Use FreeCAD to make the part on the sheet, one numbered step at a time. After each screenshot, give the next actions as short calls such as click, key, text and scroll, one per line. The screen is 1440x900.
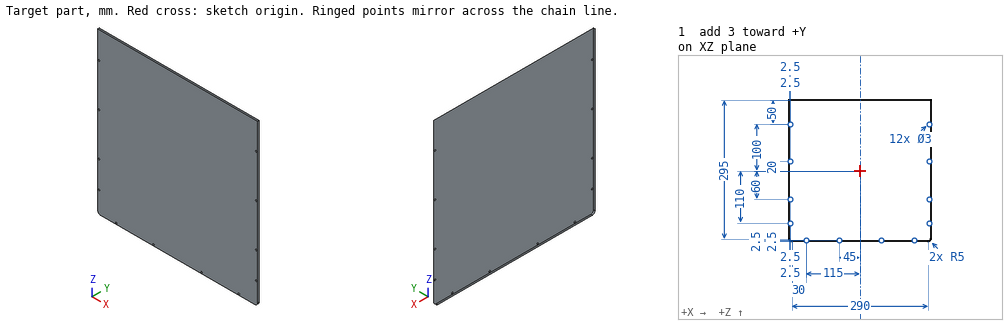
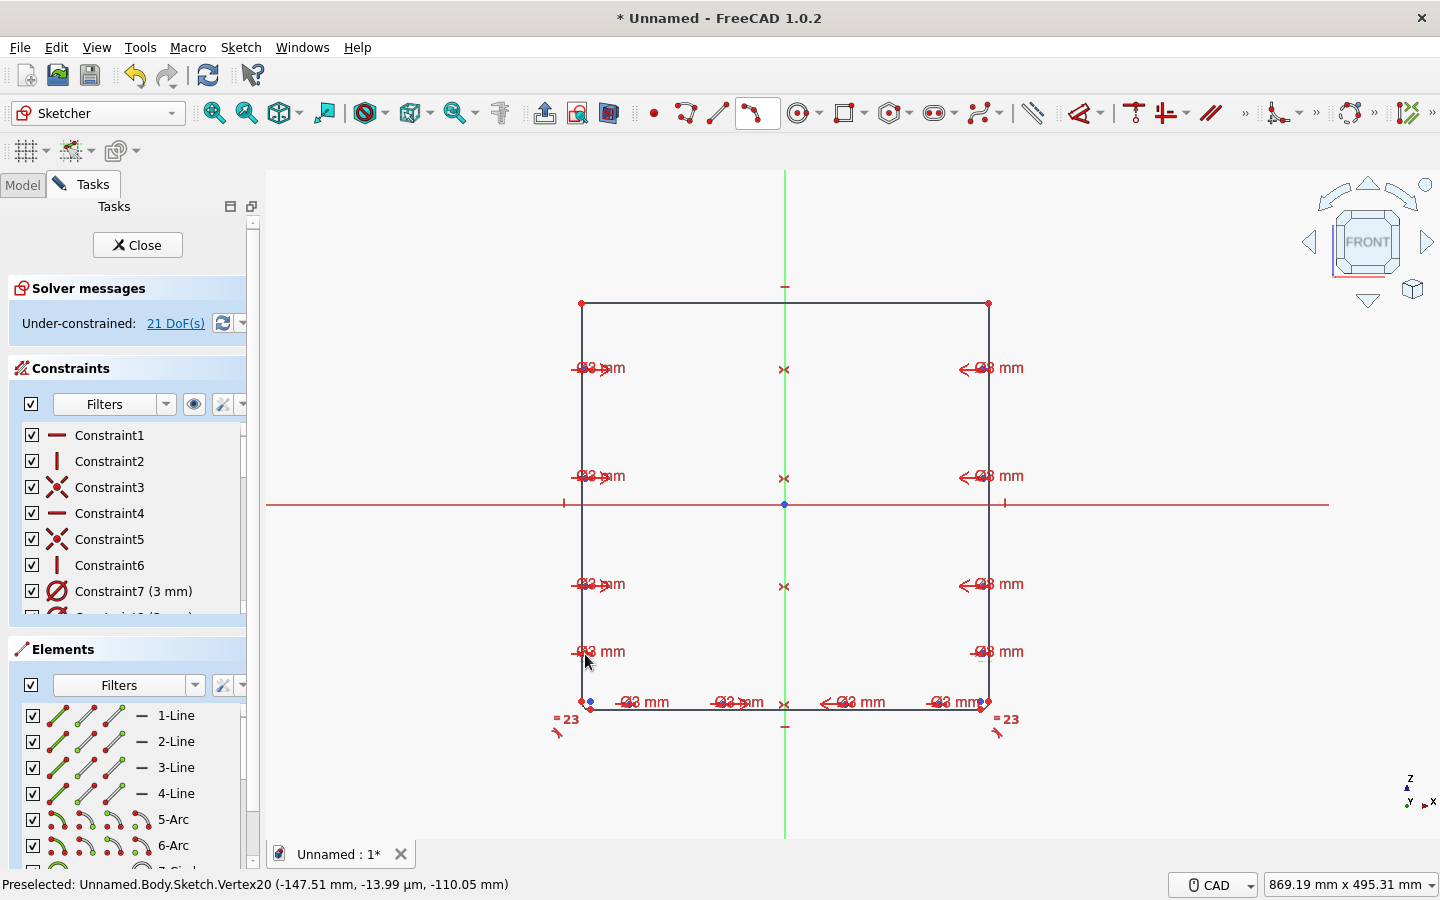
click(984, 654)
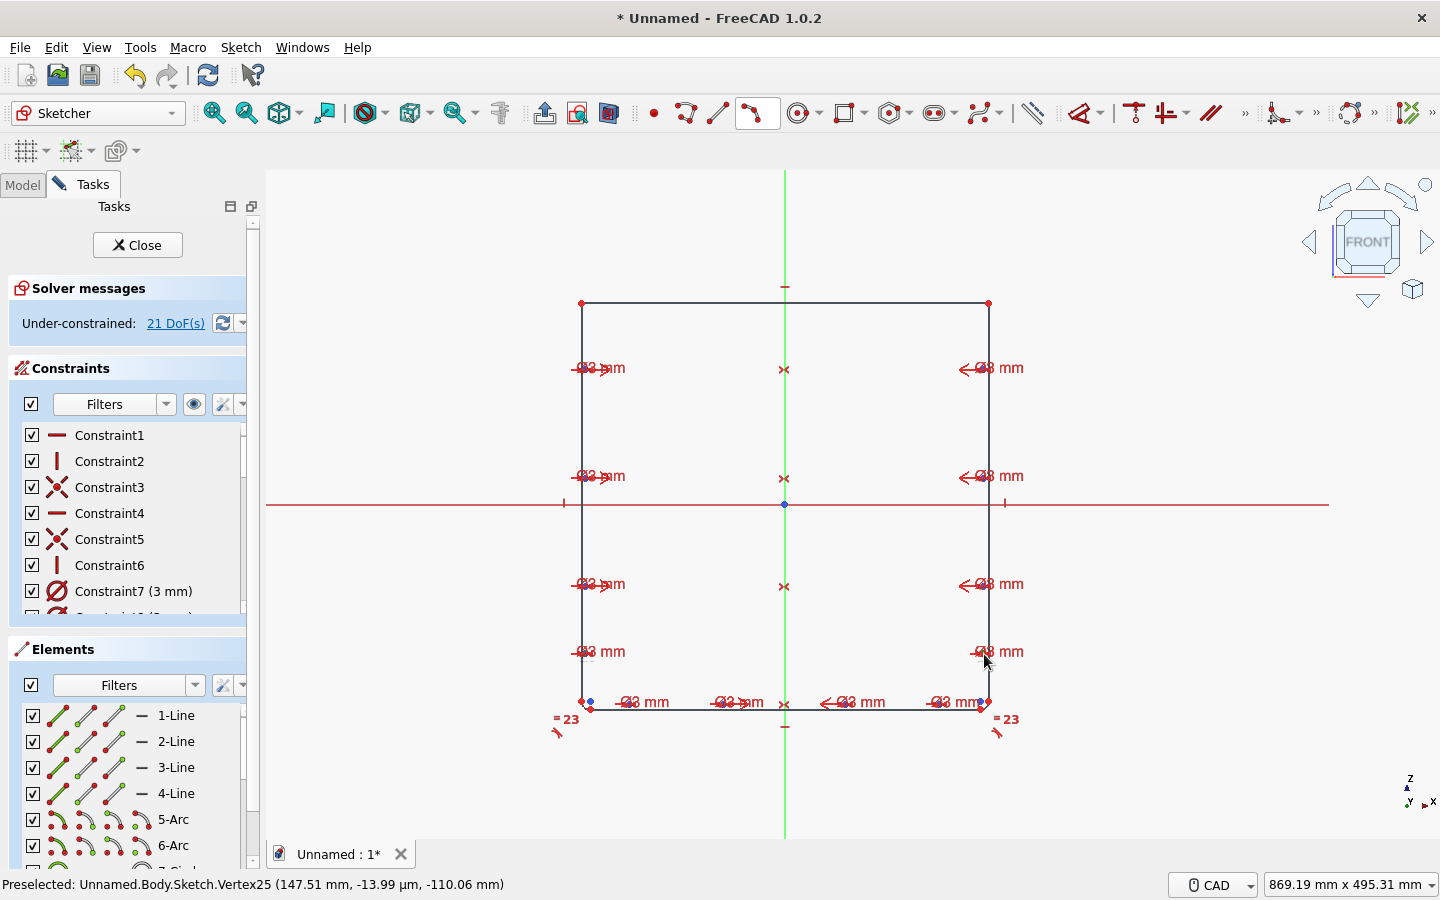
click(785, 767)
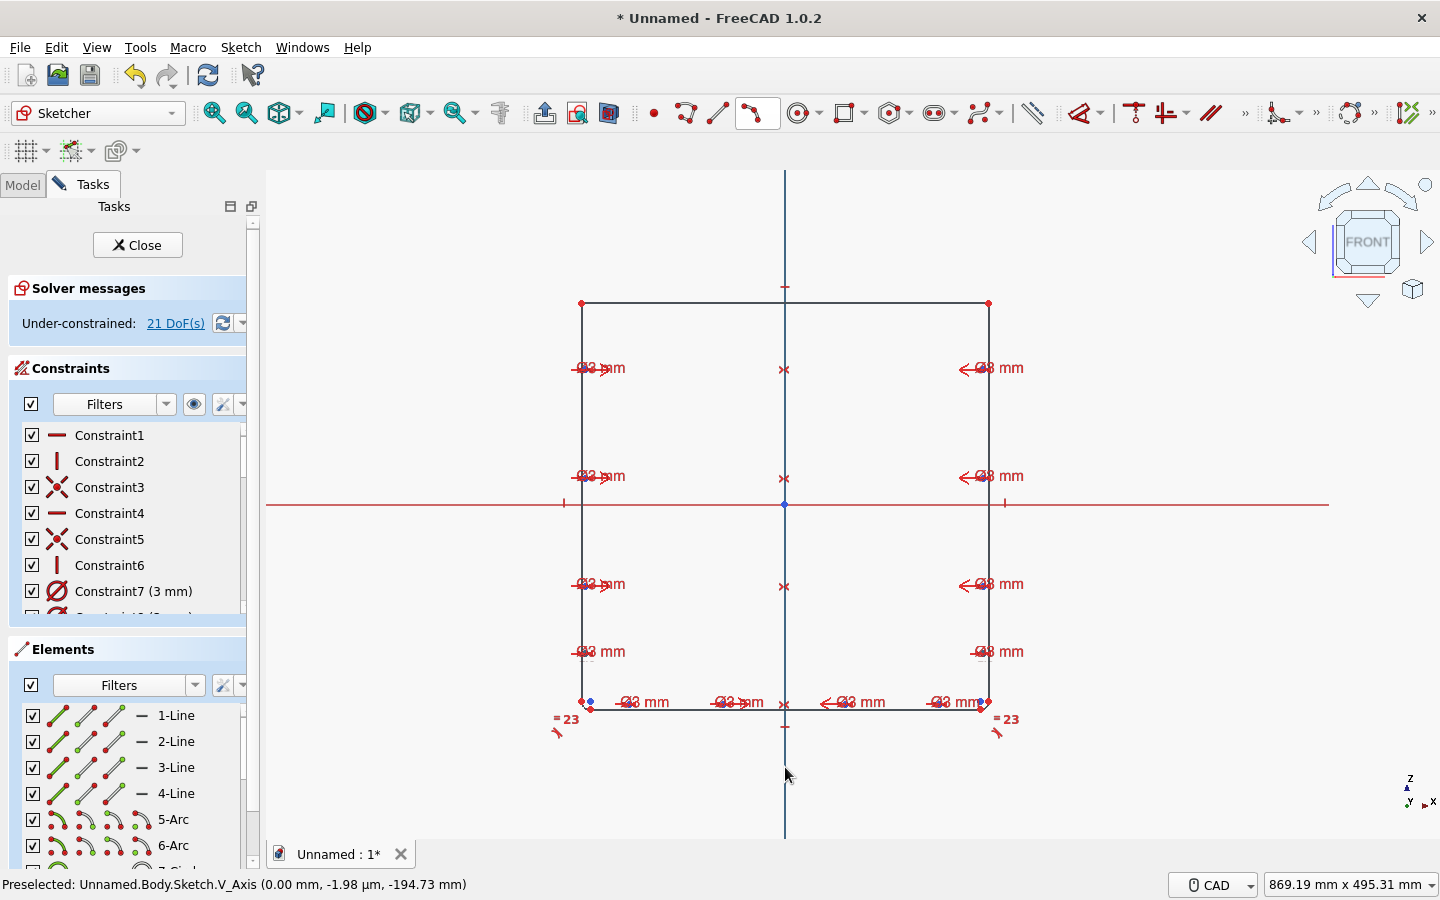
key(s)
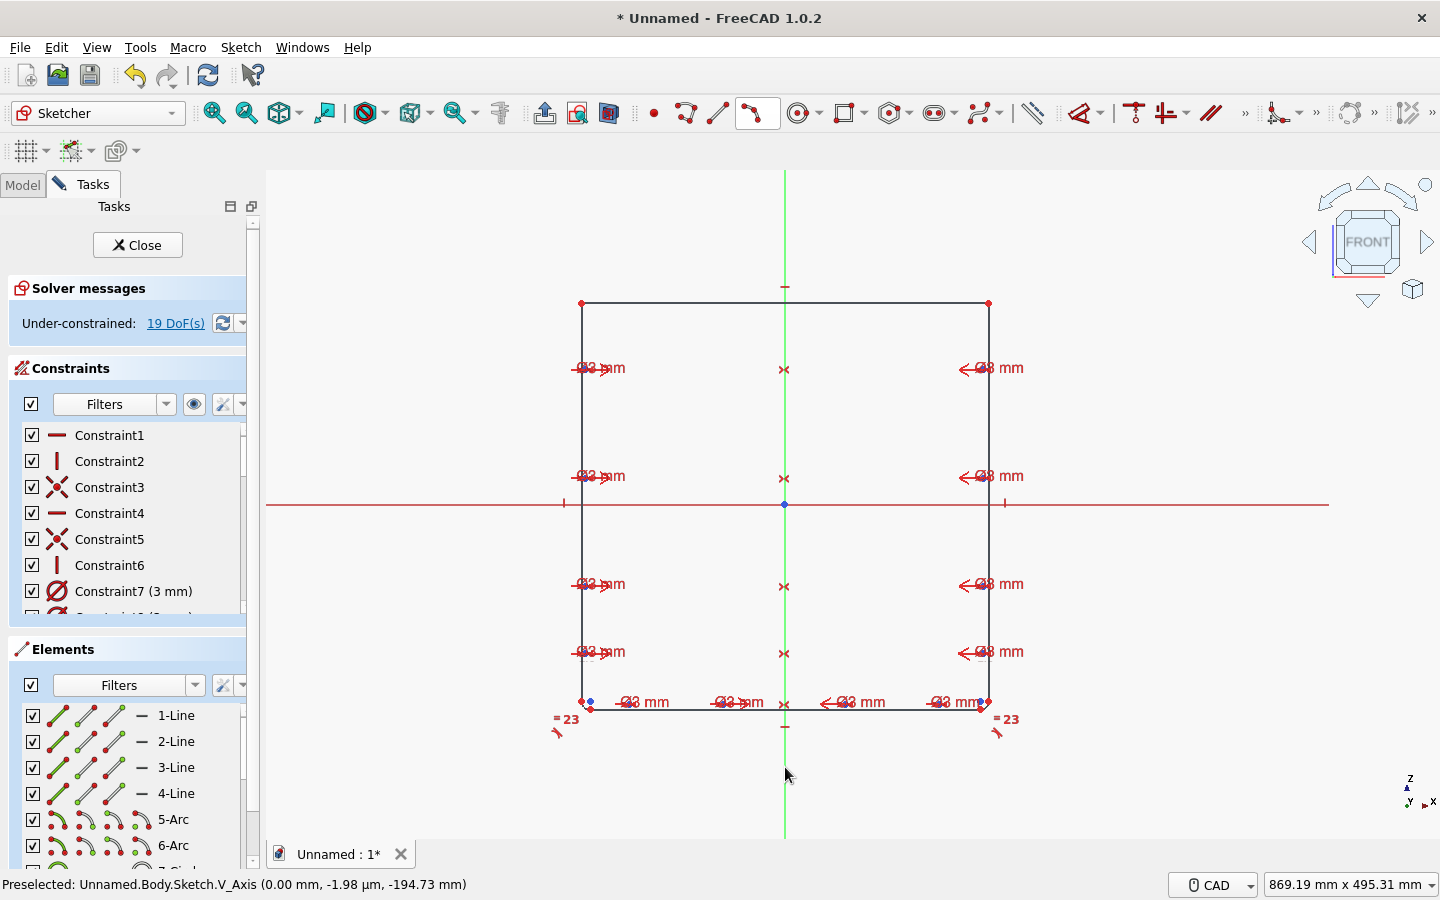
click(629, 704)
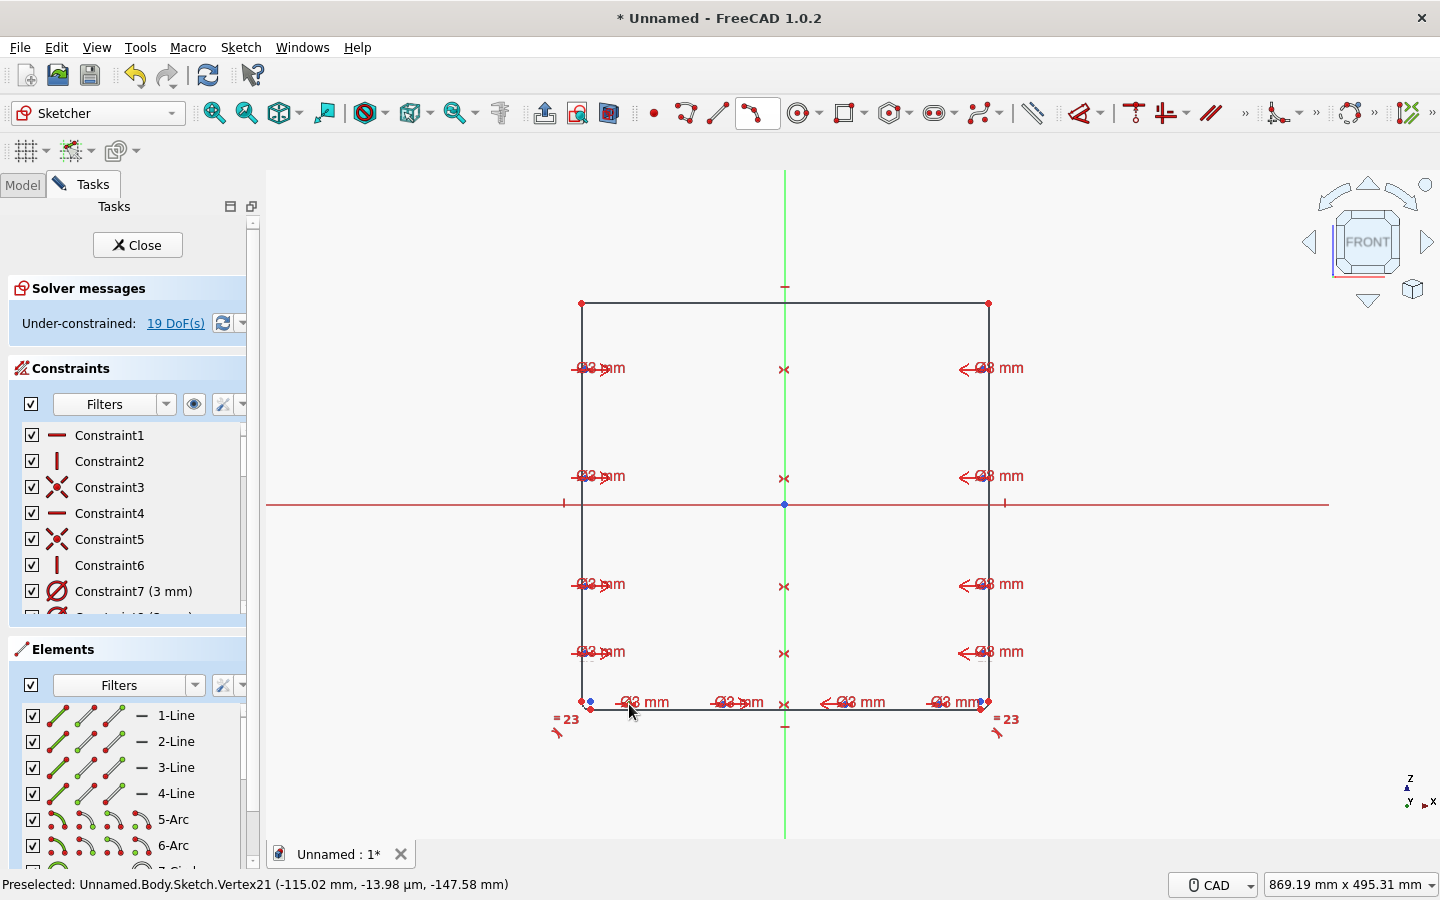
click(940, 704)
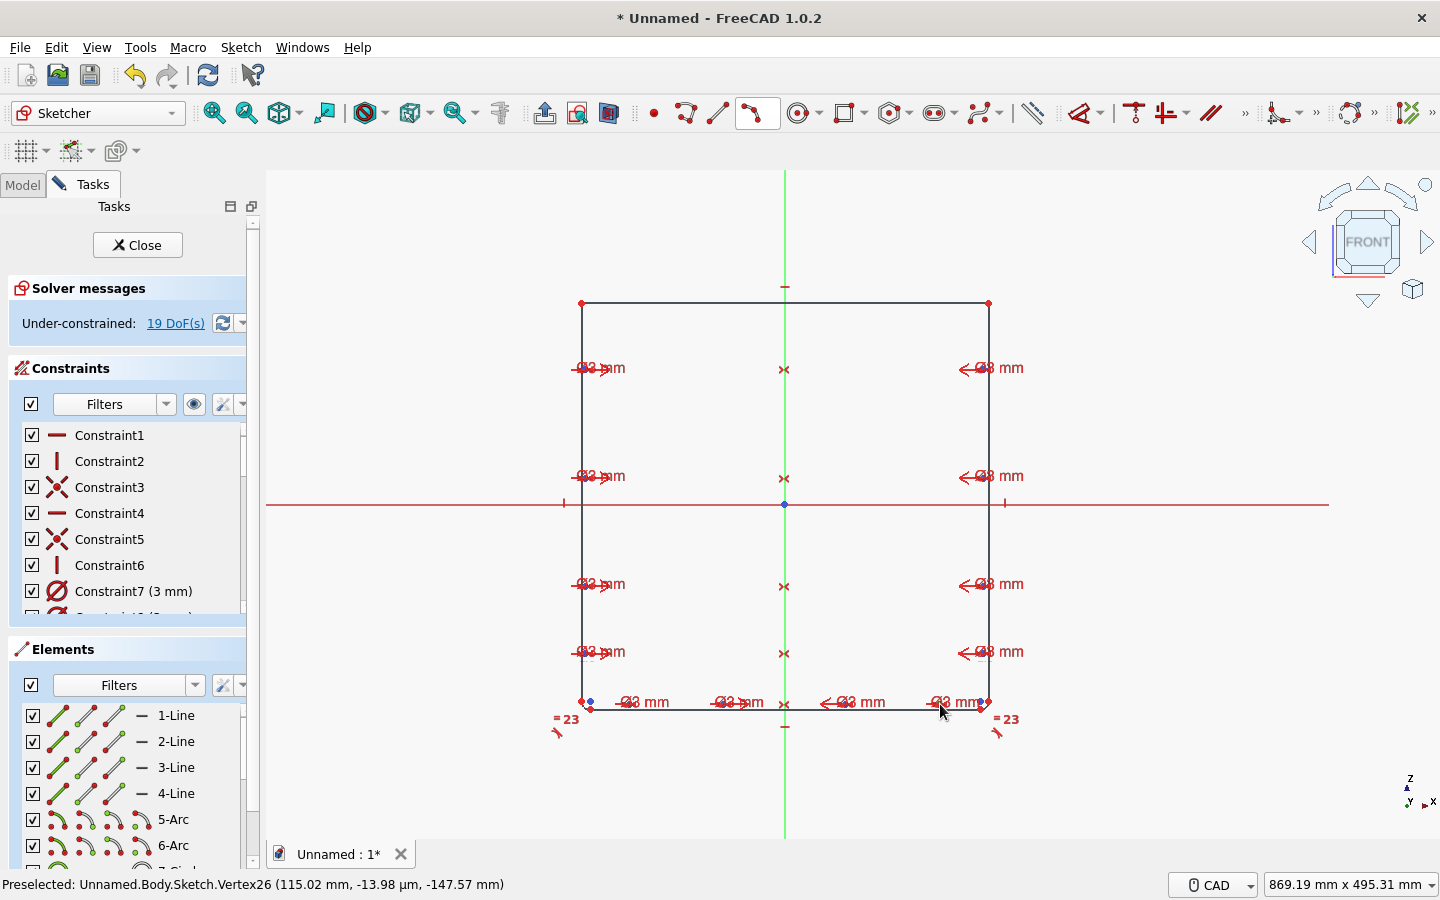
click(785, 767)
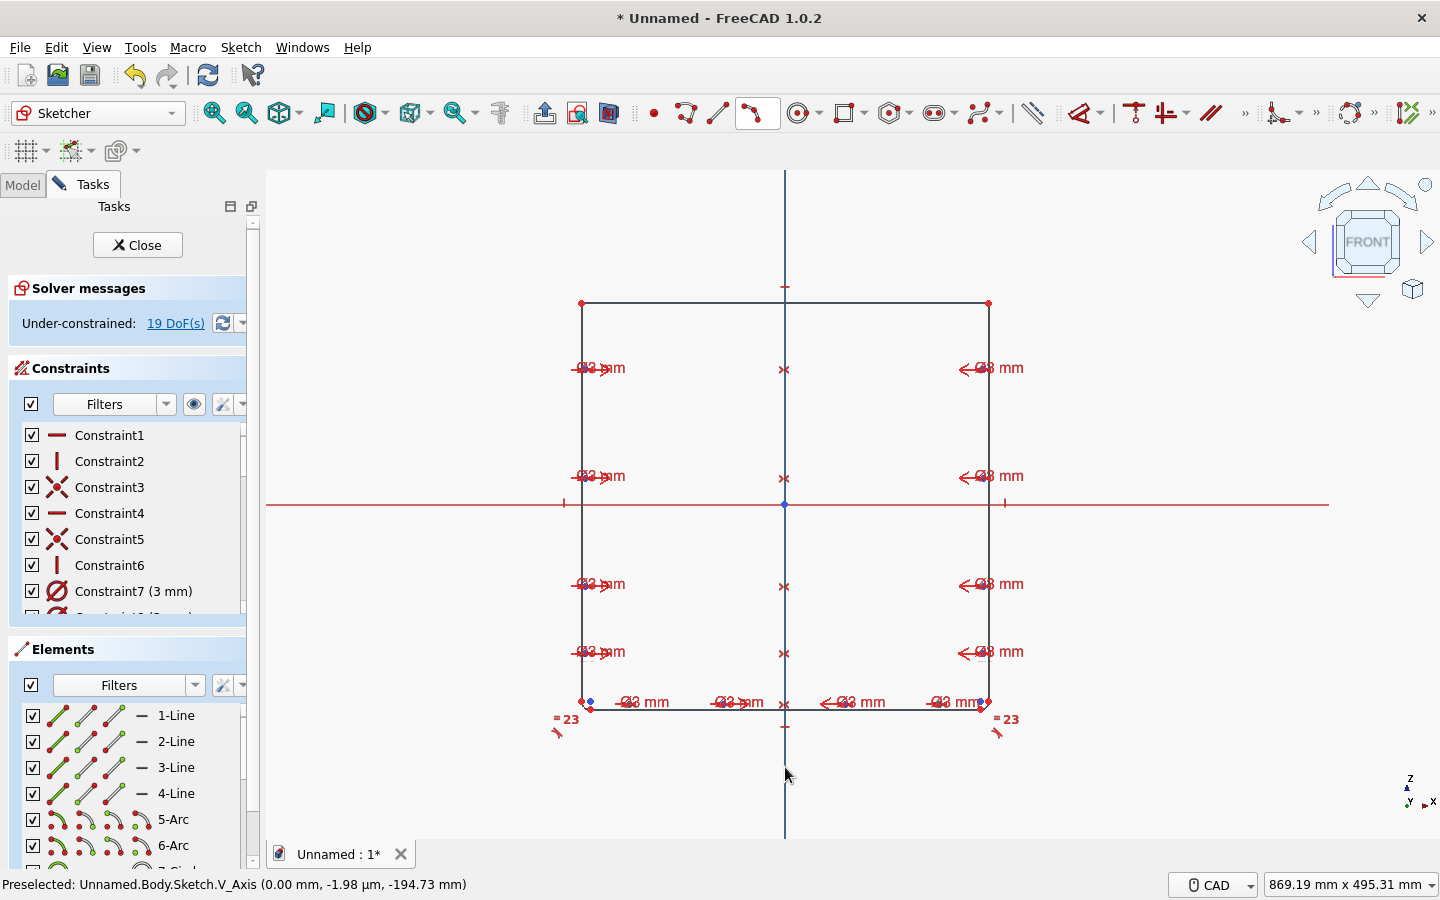
key(s)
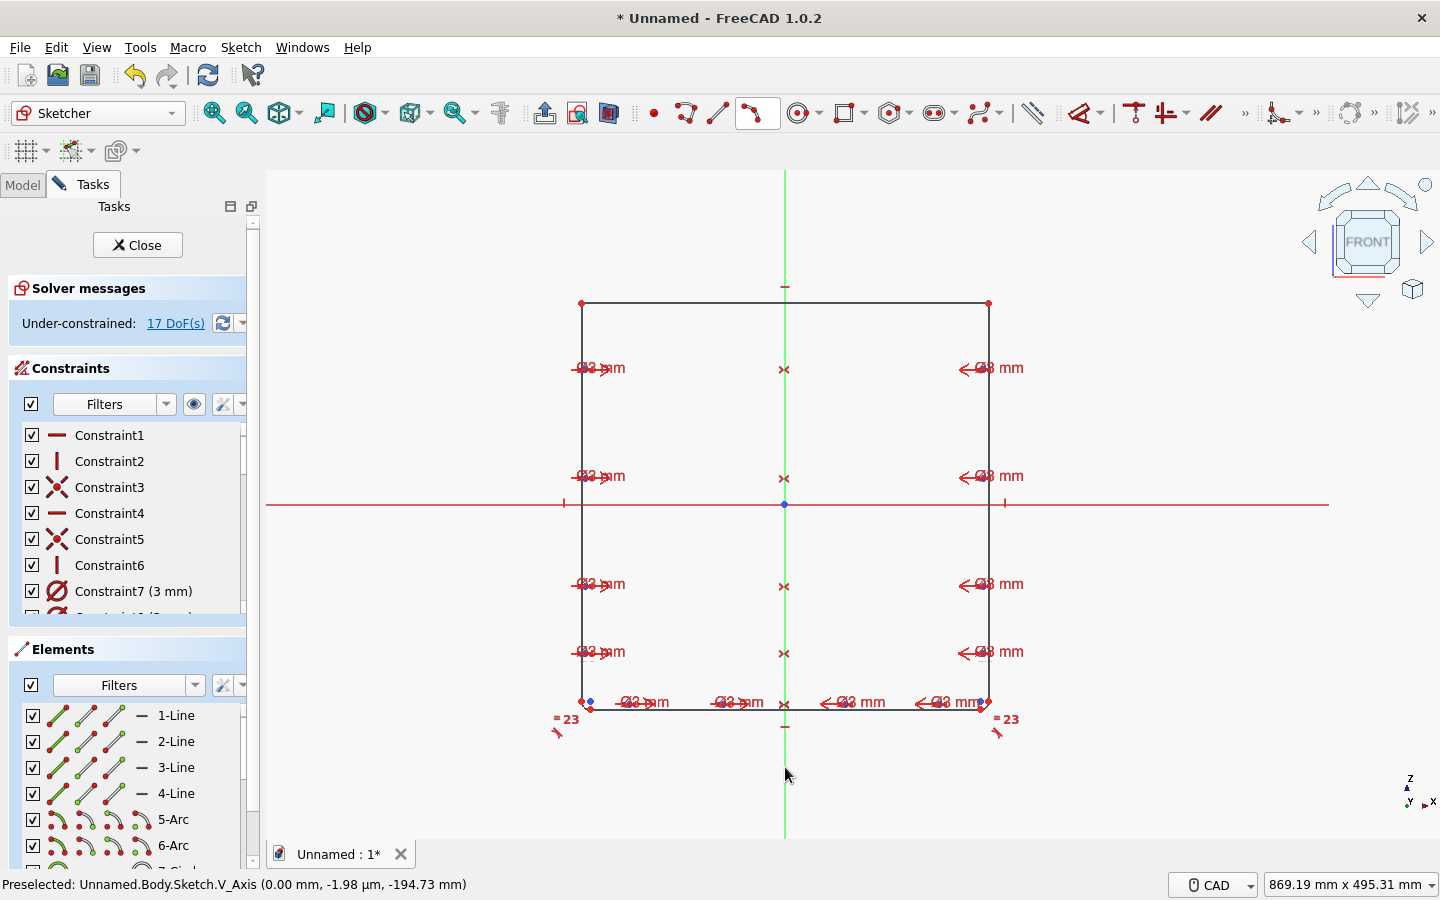
click(1080, 114)